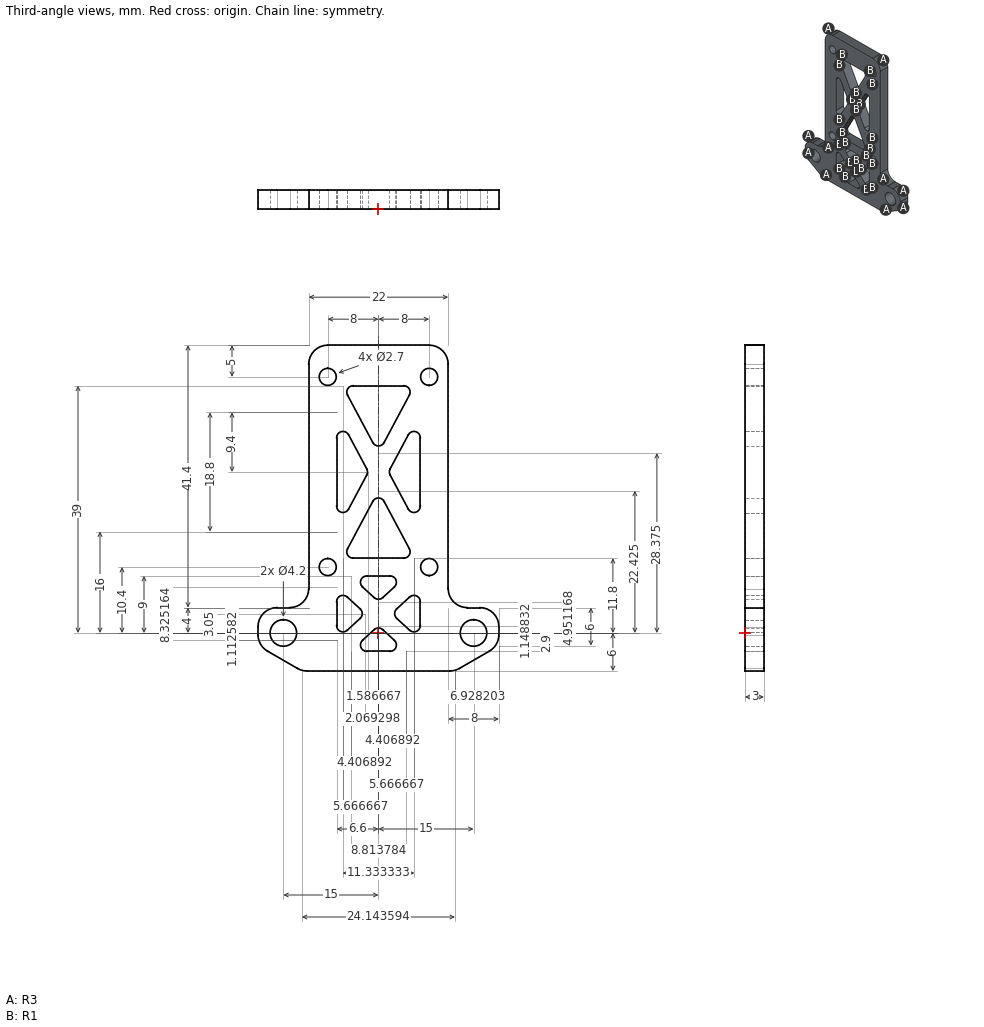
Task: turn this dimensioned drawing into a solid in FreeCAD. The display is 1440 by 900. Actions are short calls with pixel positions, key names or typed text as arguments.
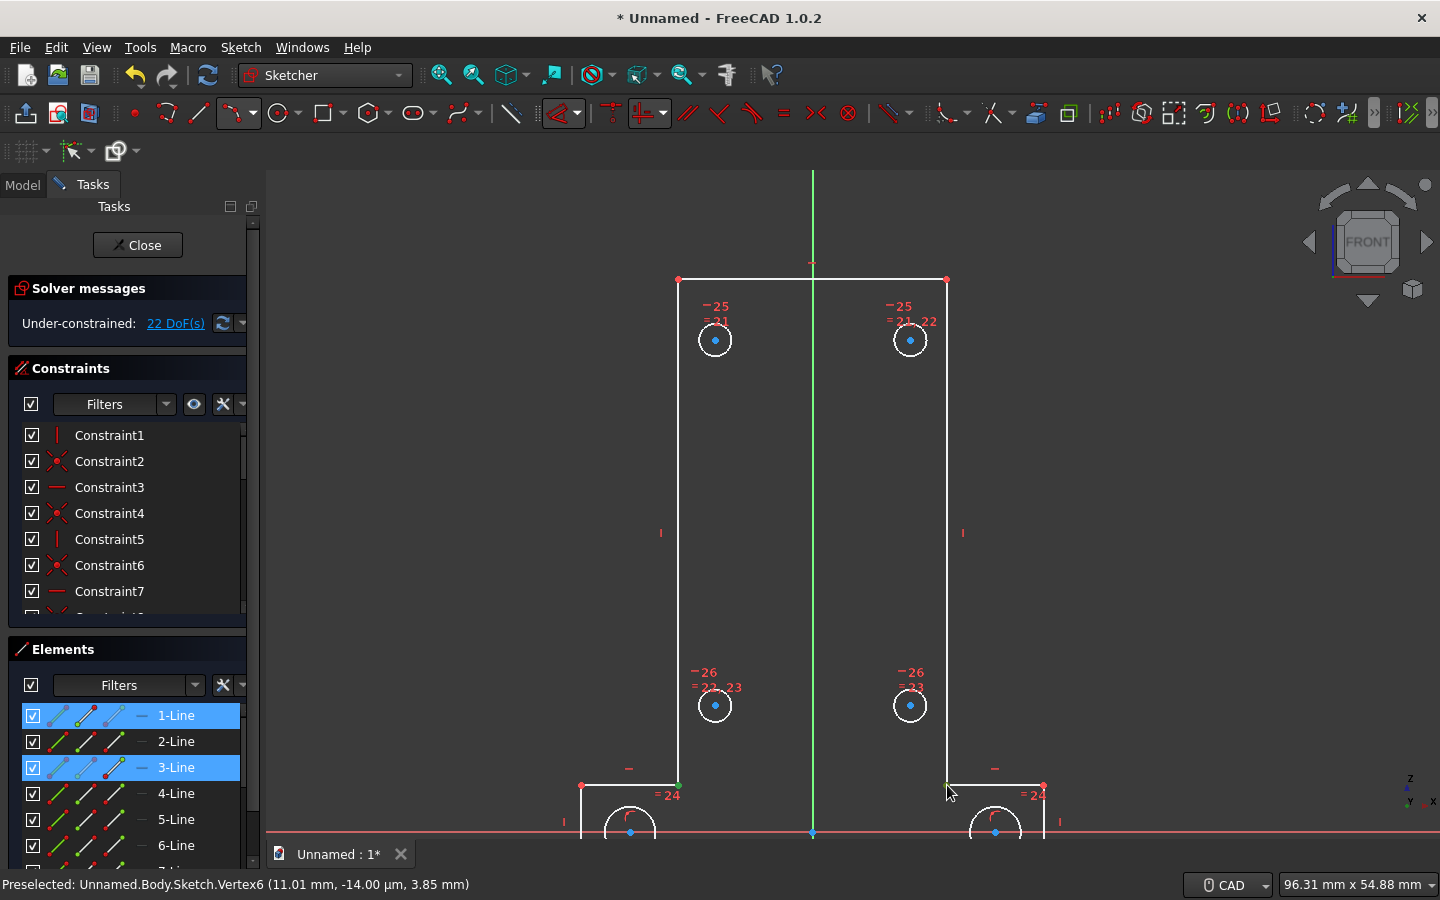
click(813, 767)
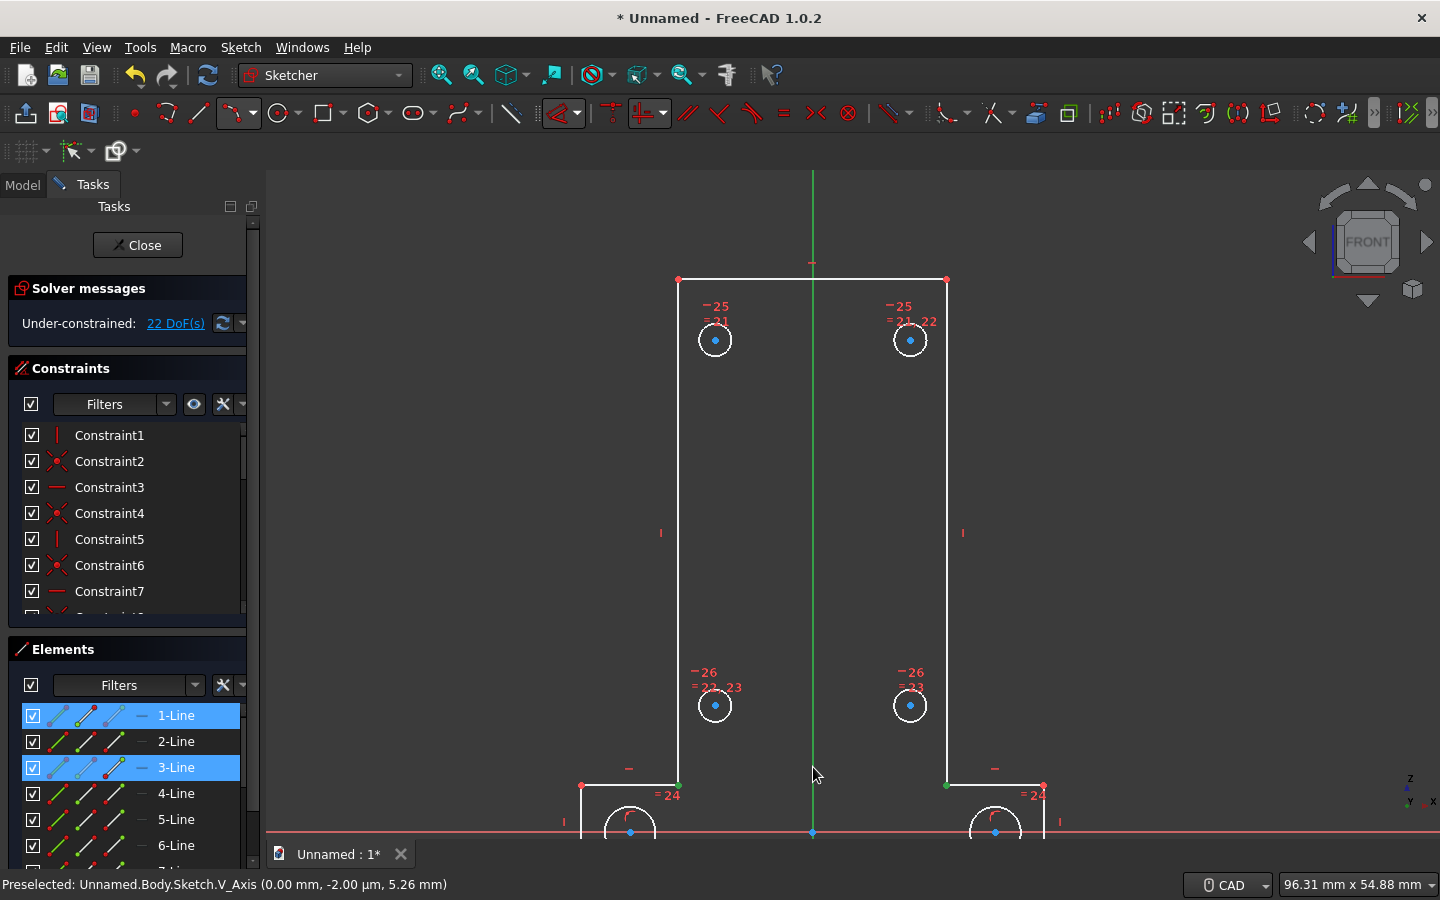
click(816, 114)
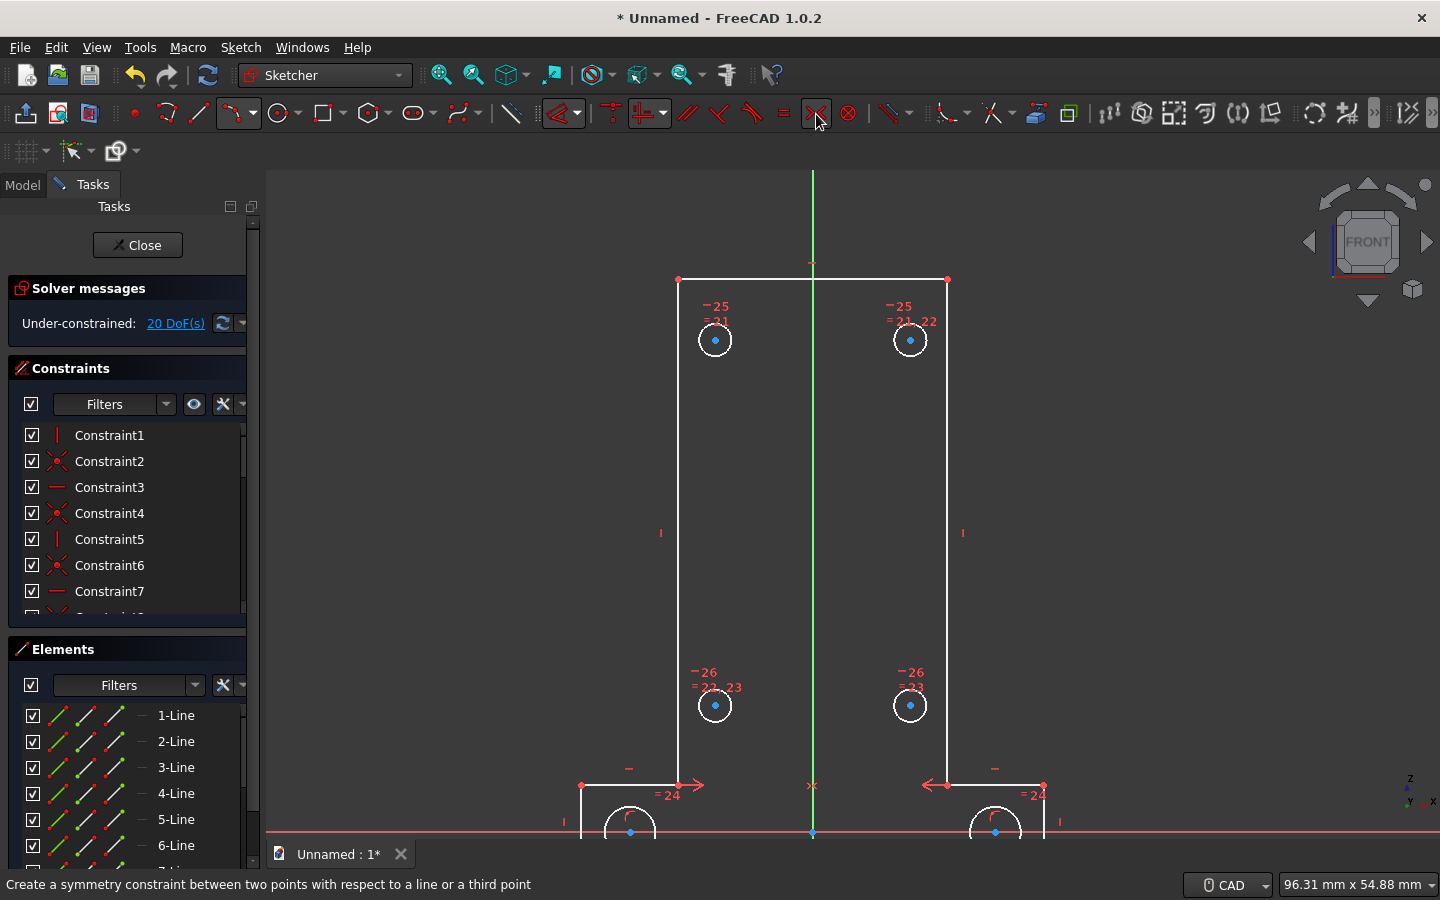
scroll(727, 327, down, 2)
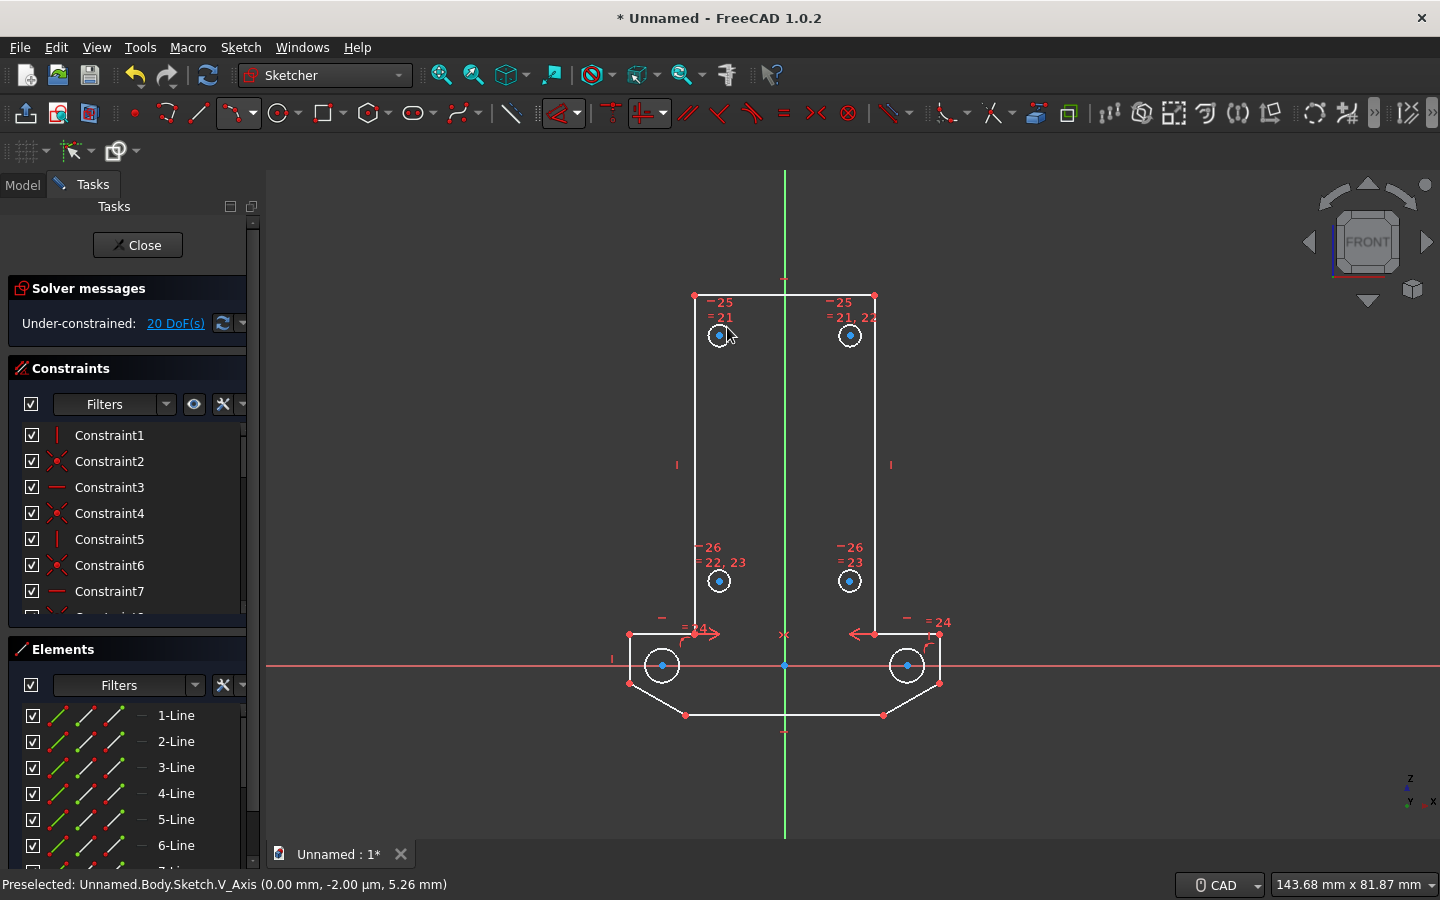
click(940, 683)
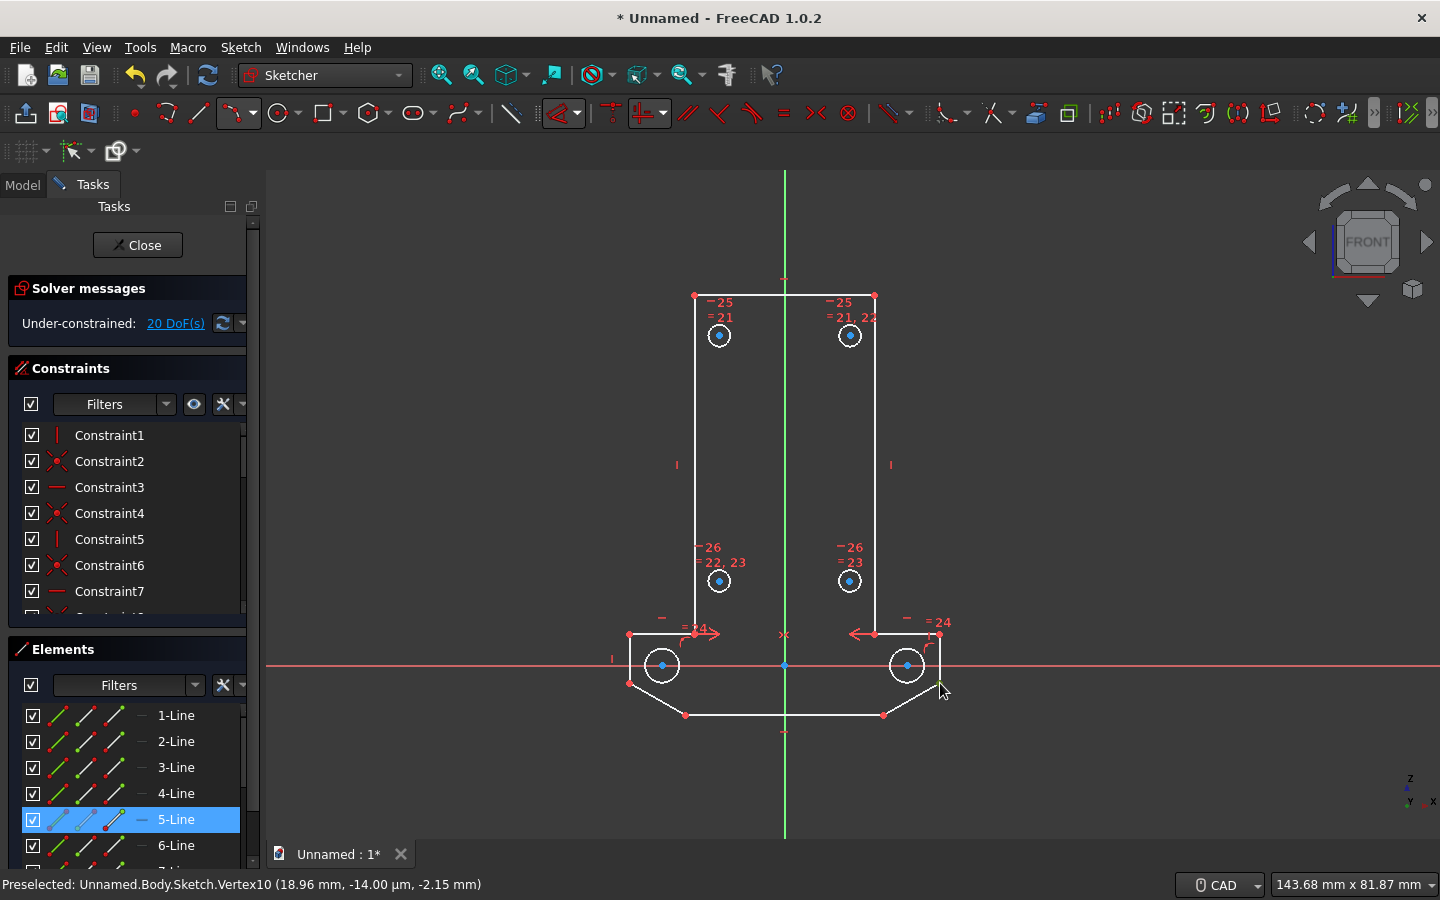
click(630, 683)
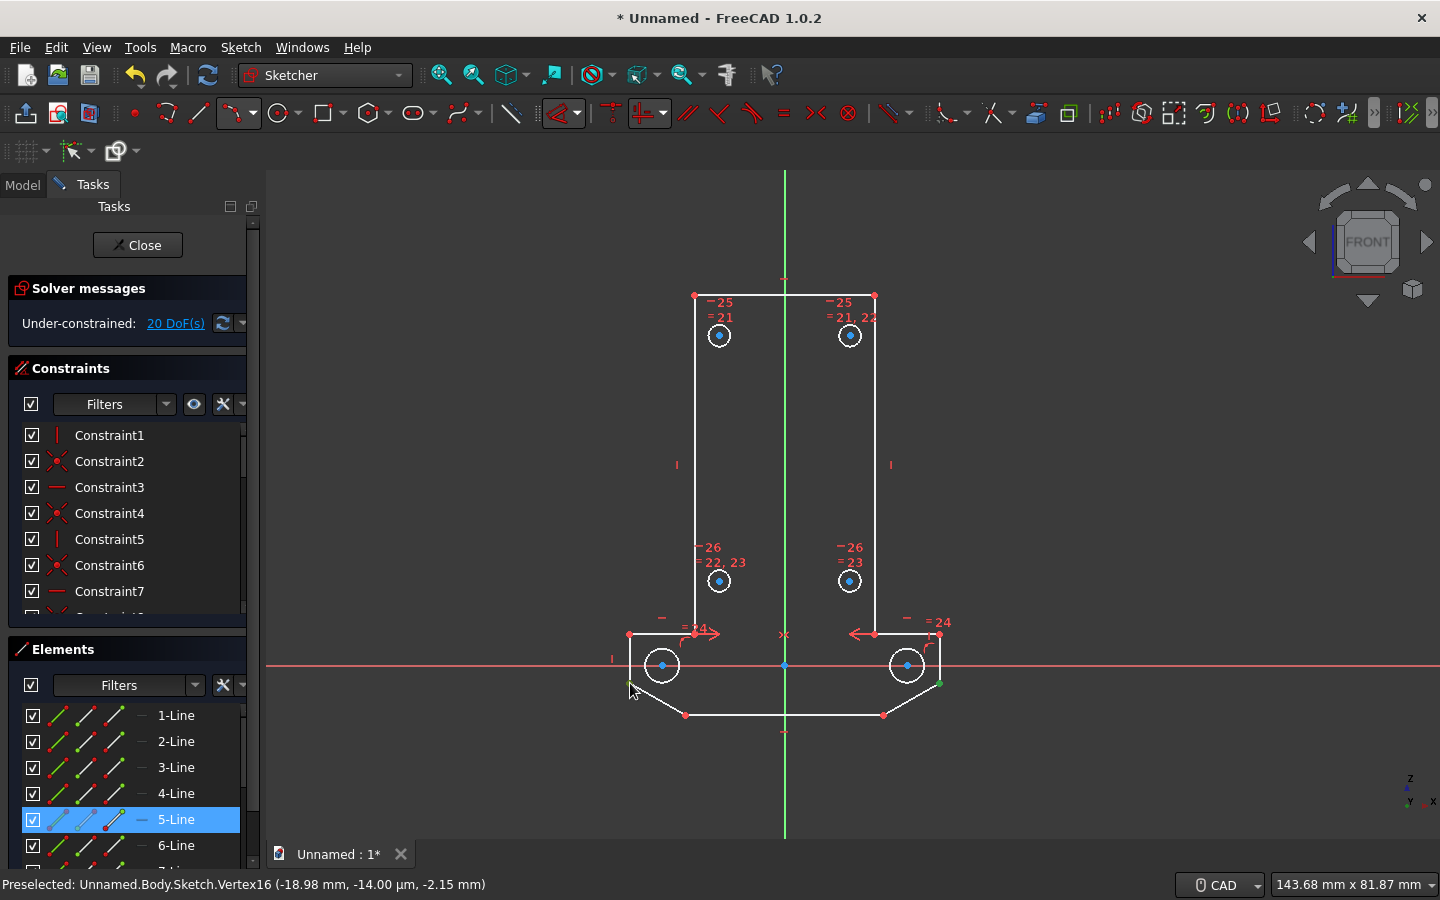
click(785, 767)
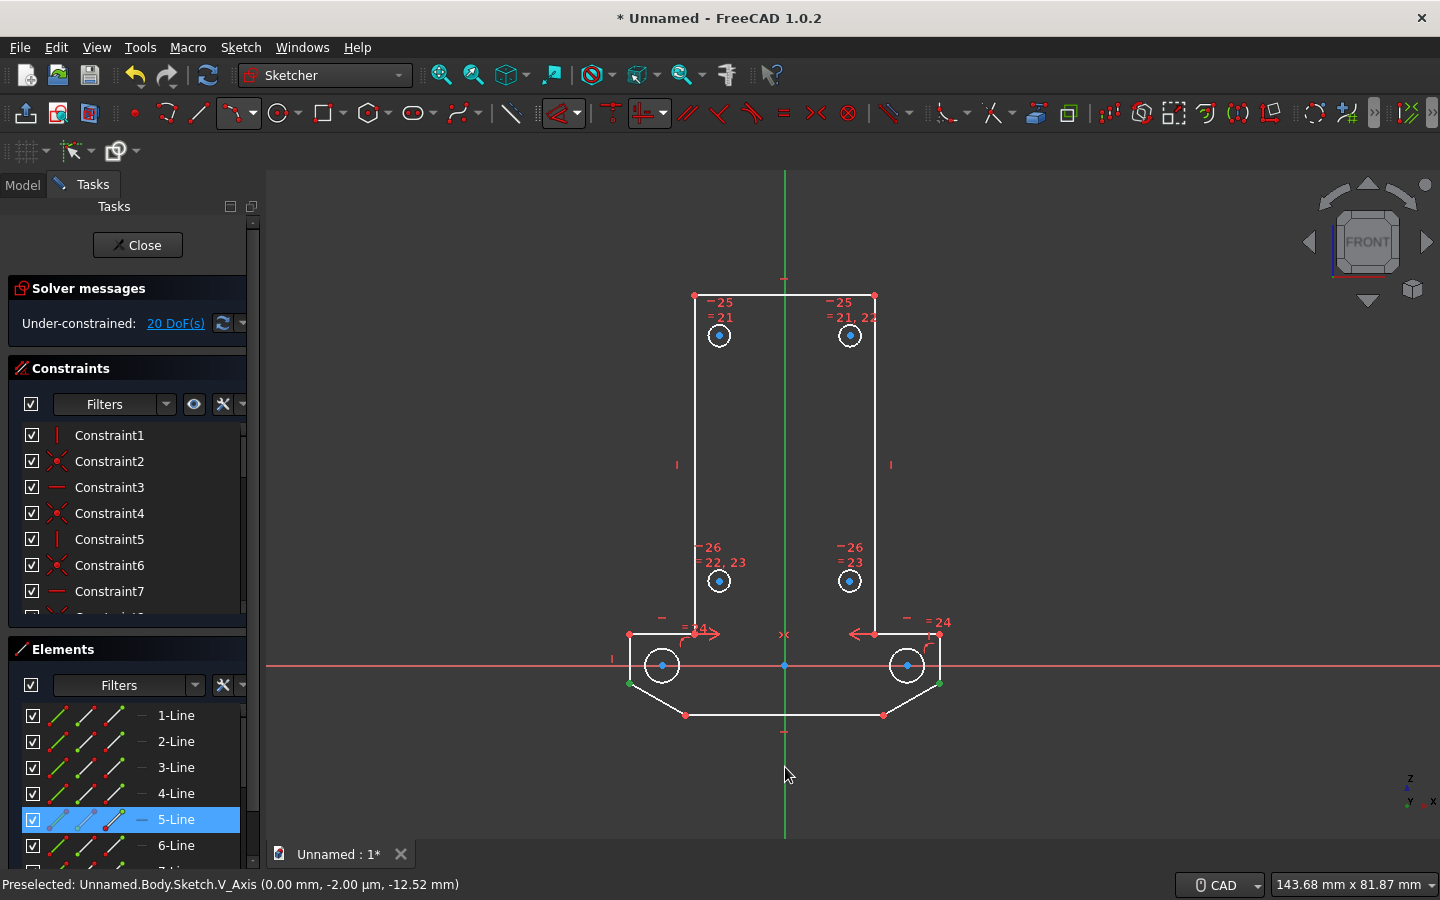
click(816, 114)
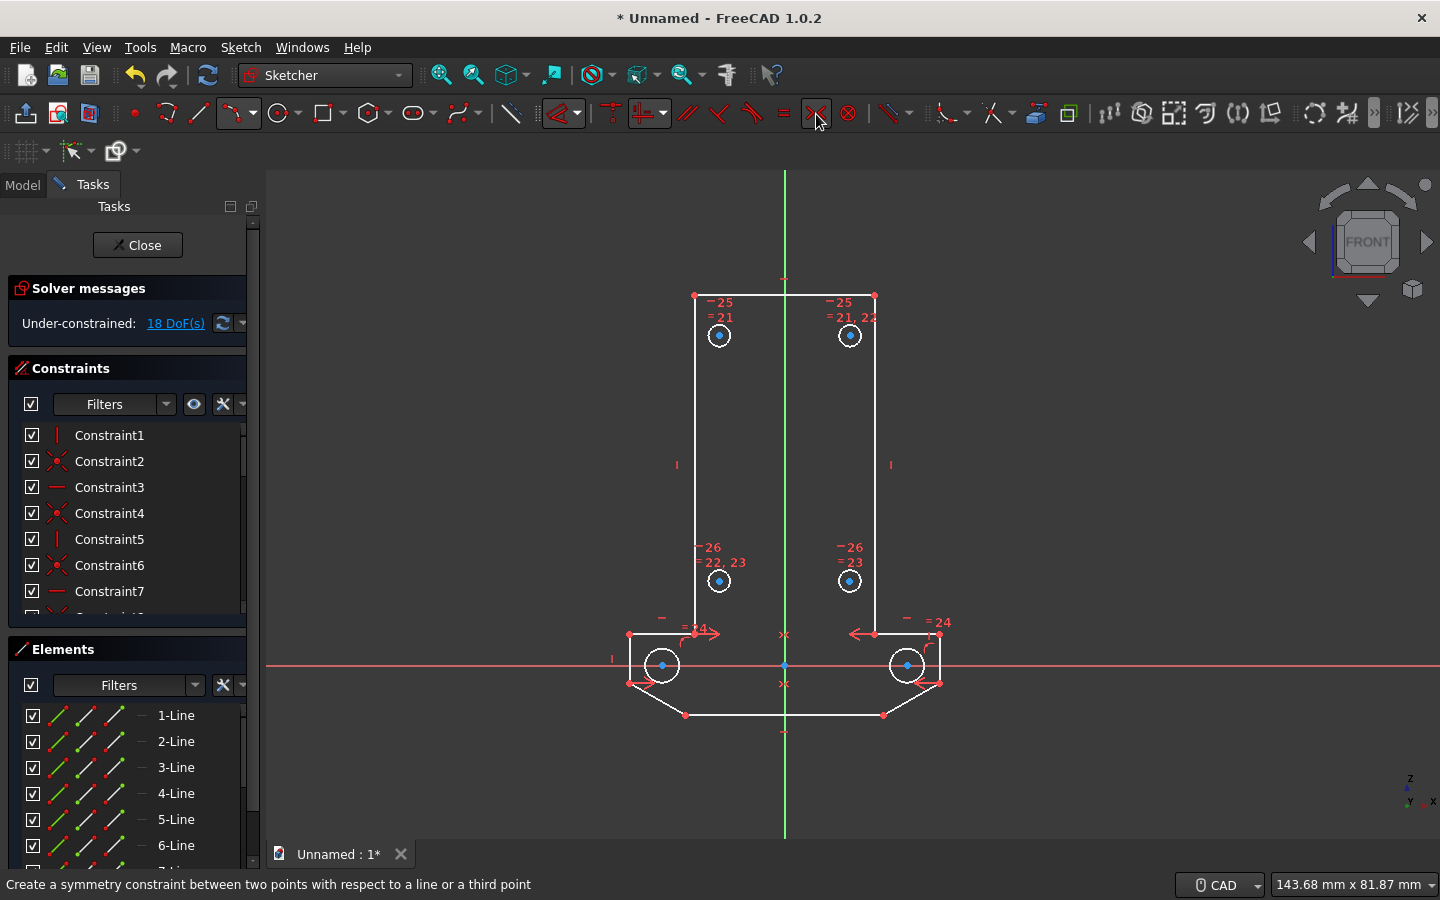
key(d)